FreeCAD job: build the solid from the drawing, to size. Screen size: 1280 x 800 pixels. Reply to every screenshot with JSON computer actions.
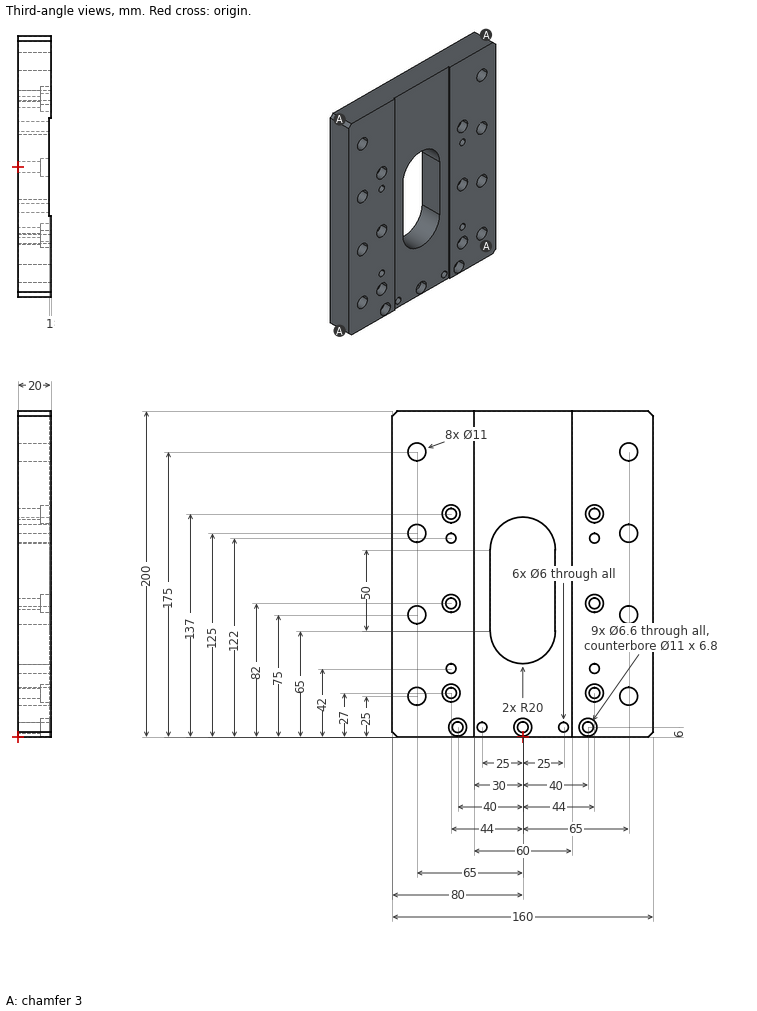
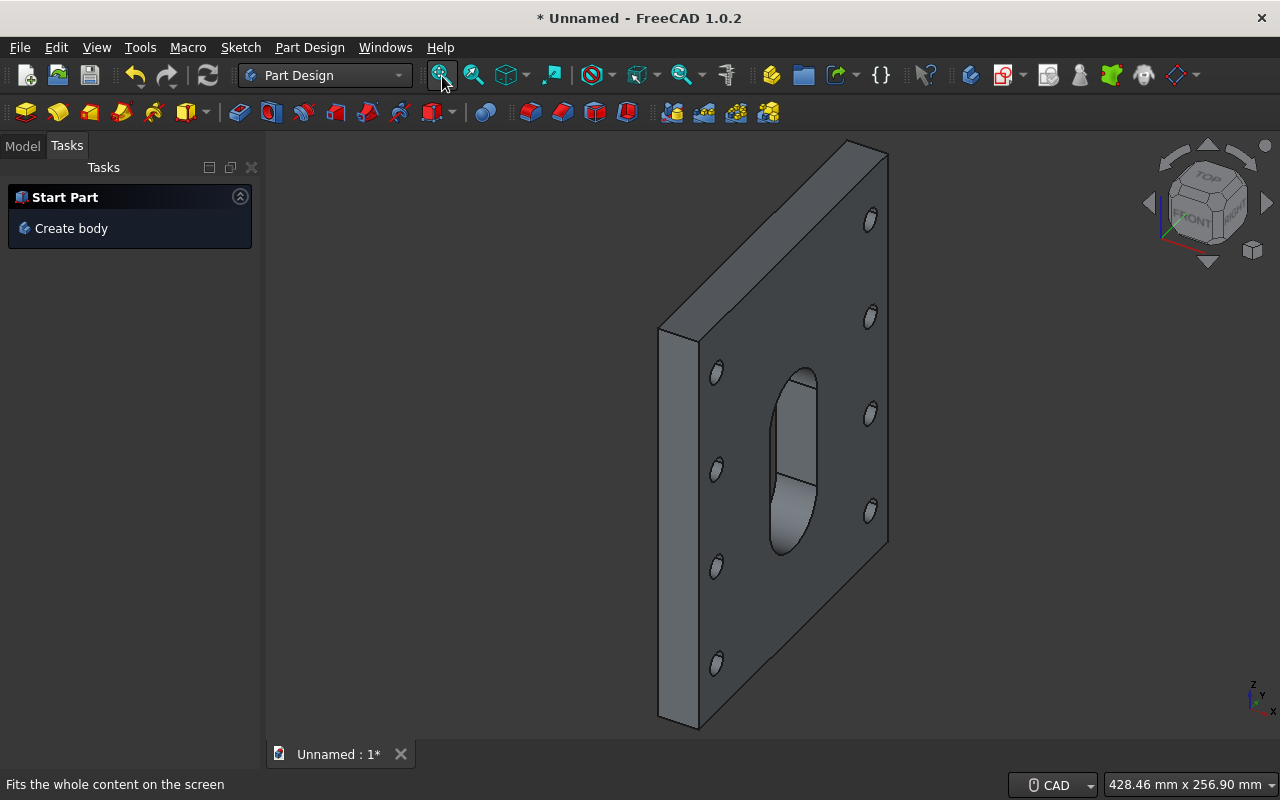
{"action": "left_click", "coordinate": [821, 303]}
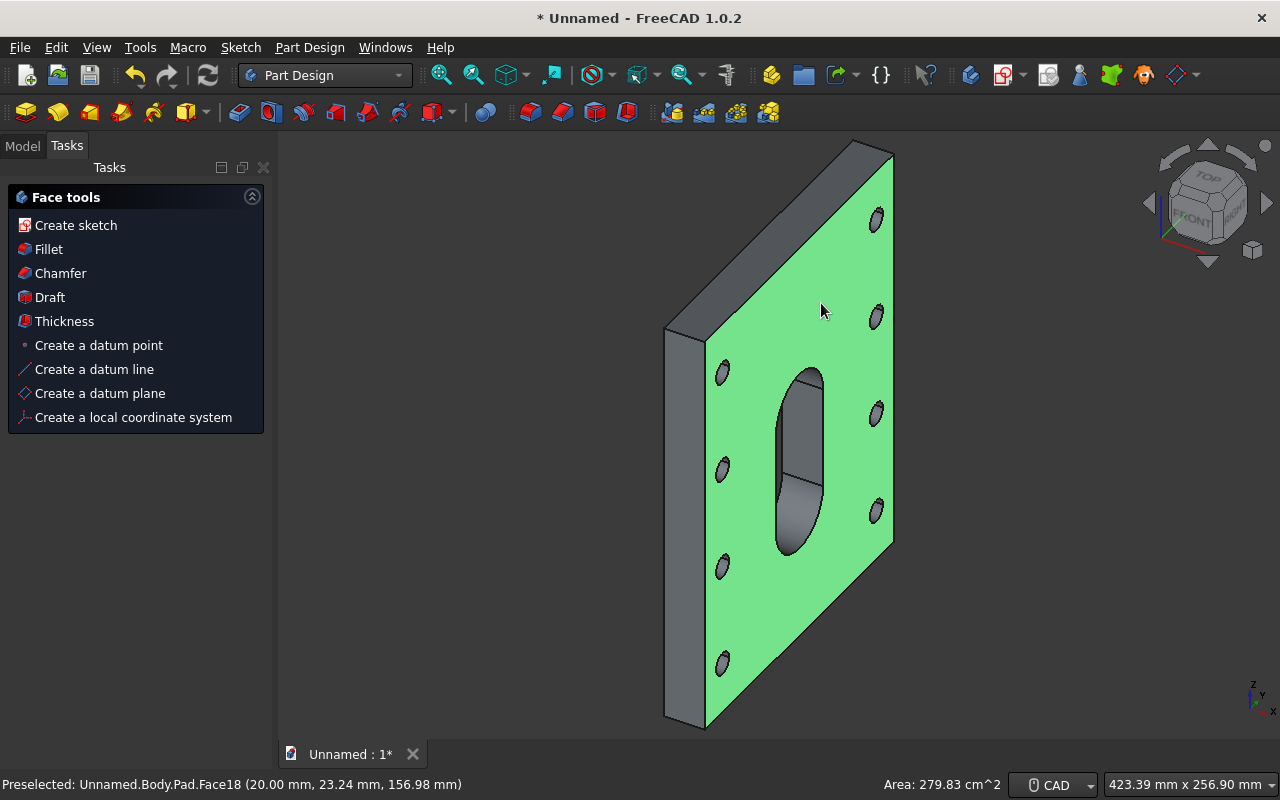
{"action": "left_click", "coordinate": [1004, 76]}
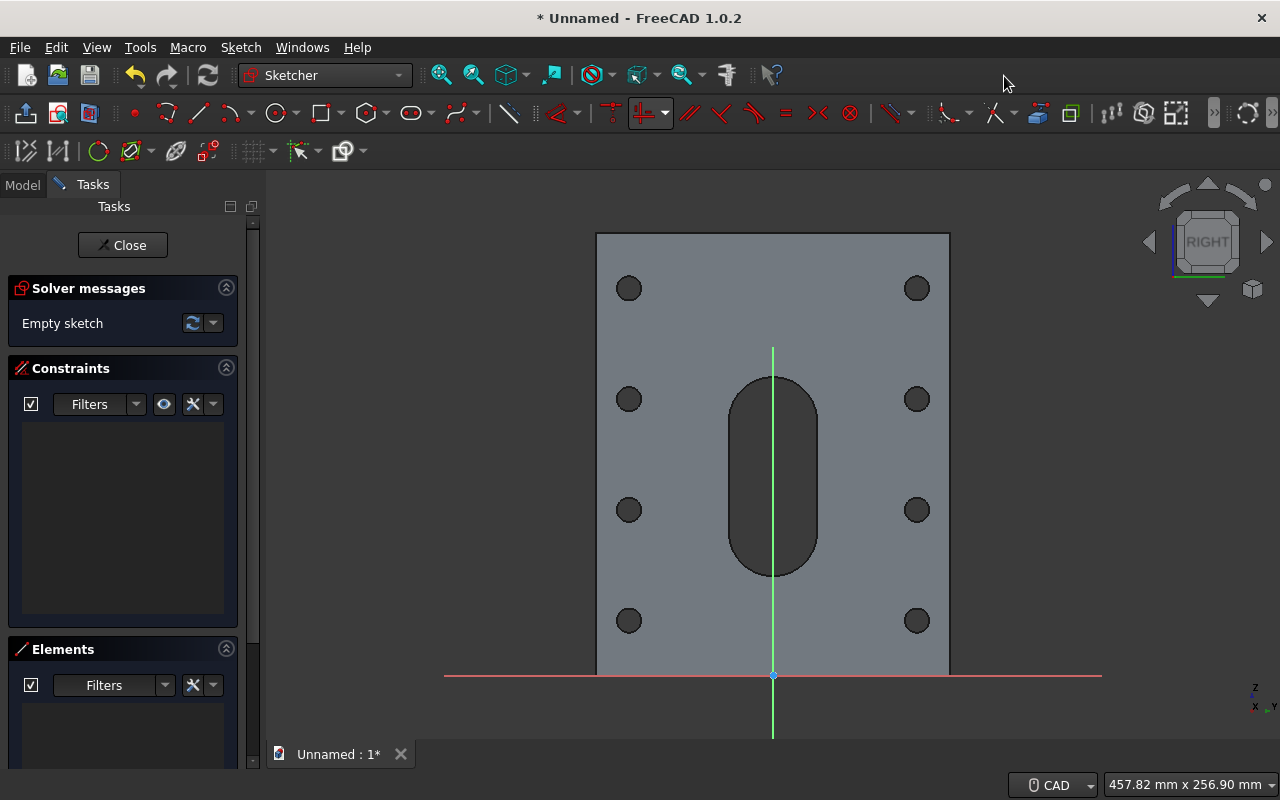
{"action": "key", "text": "g c"}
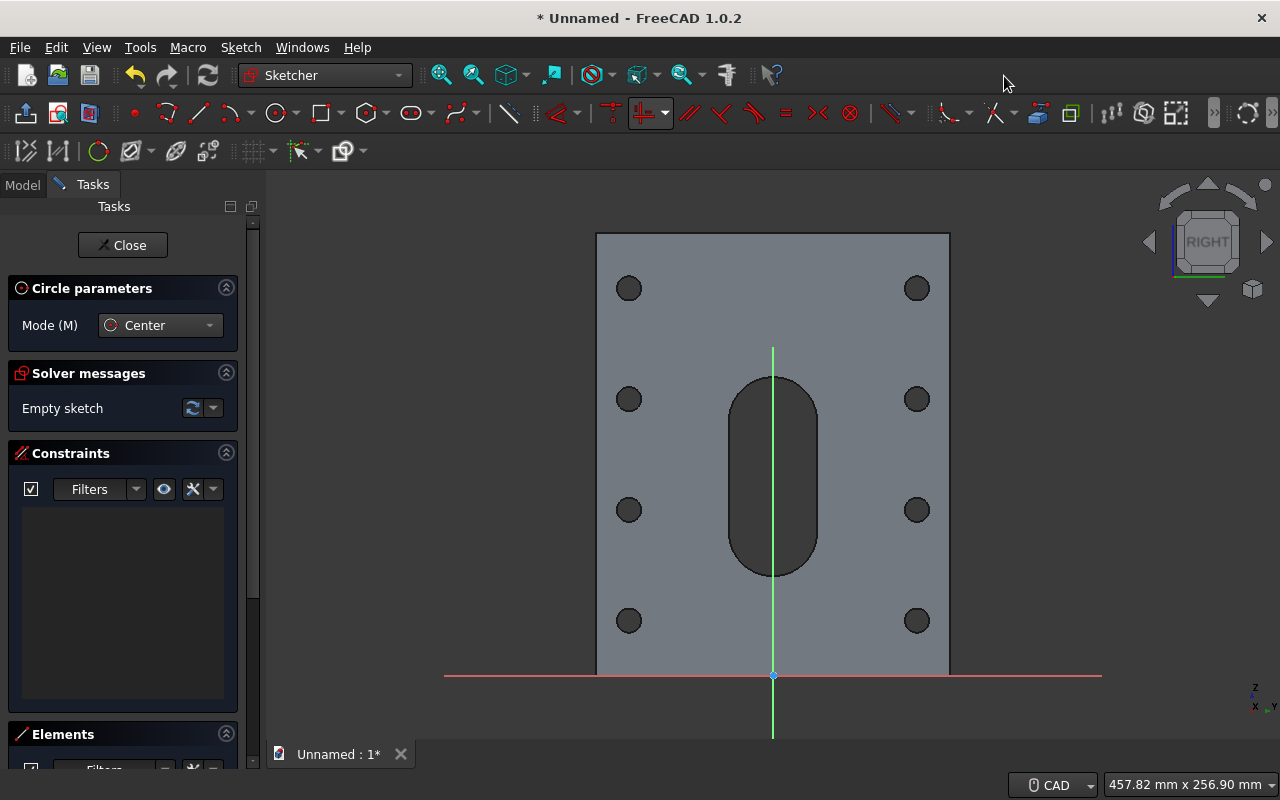
{"action": "scroll", "coordinate": [862, 663], "scroll_direction": "up", "scroll_amount": 6}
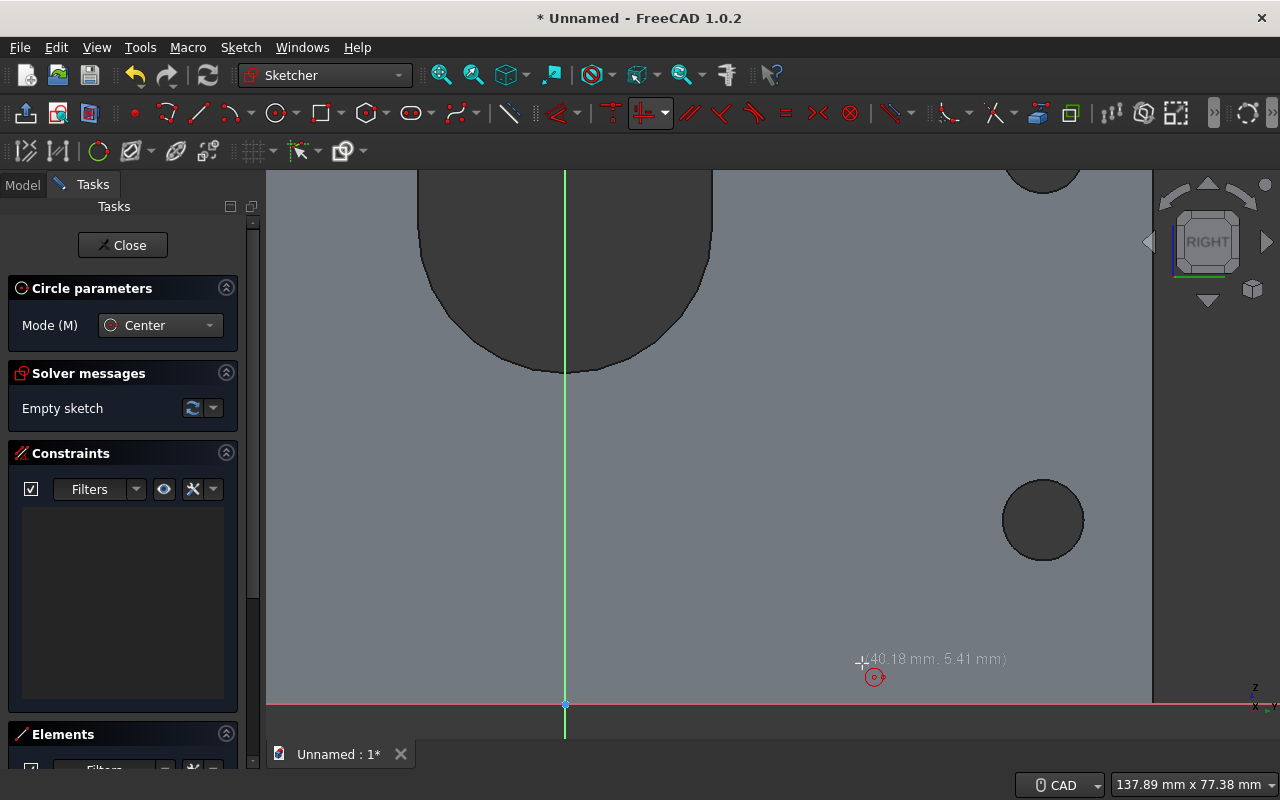
{"action": "left_click", "coordinate": [859, 660]}
{"action": "mouse_move", "coordinate": [876, 643]}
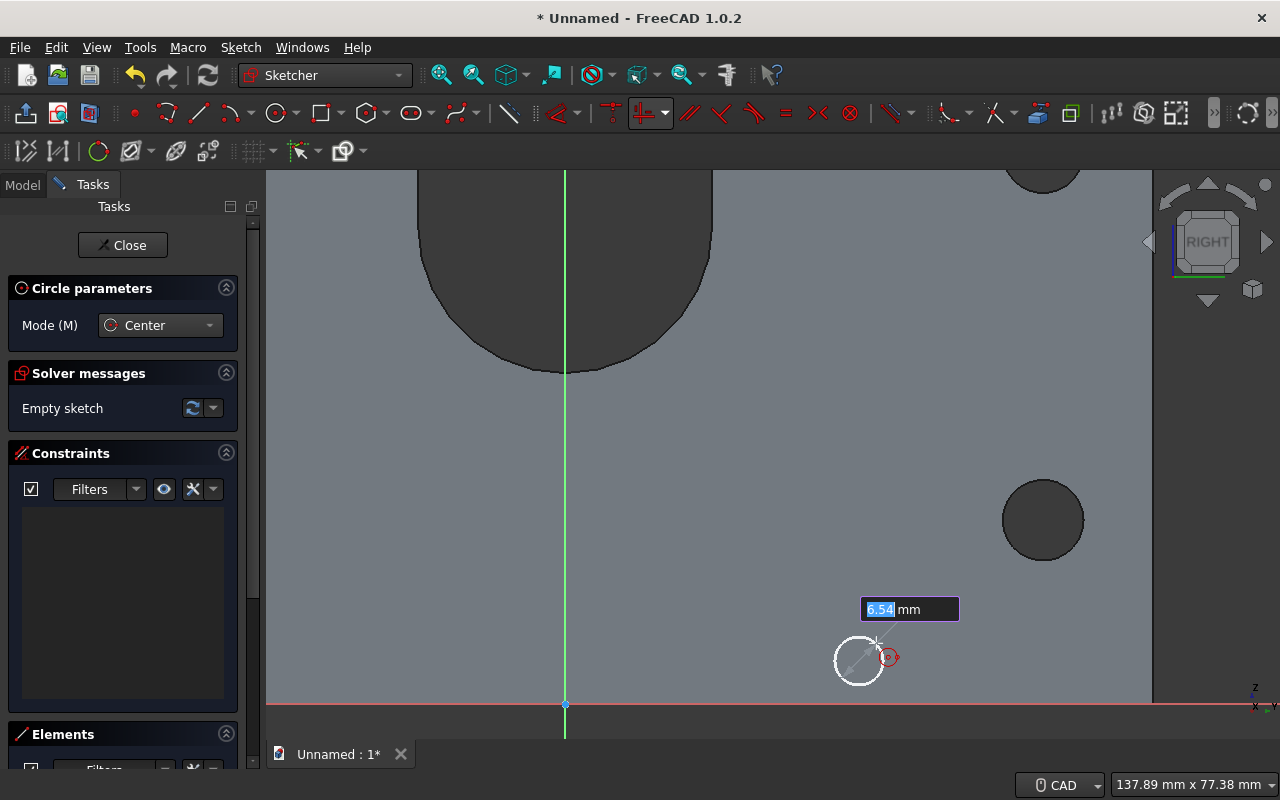
{"action": "type", "text": "6.6"}
{"action": "key", "text": "Return"}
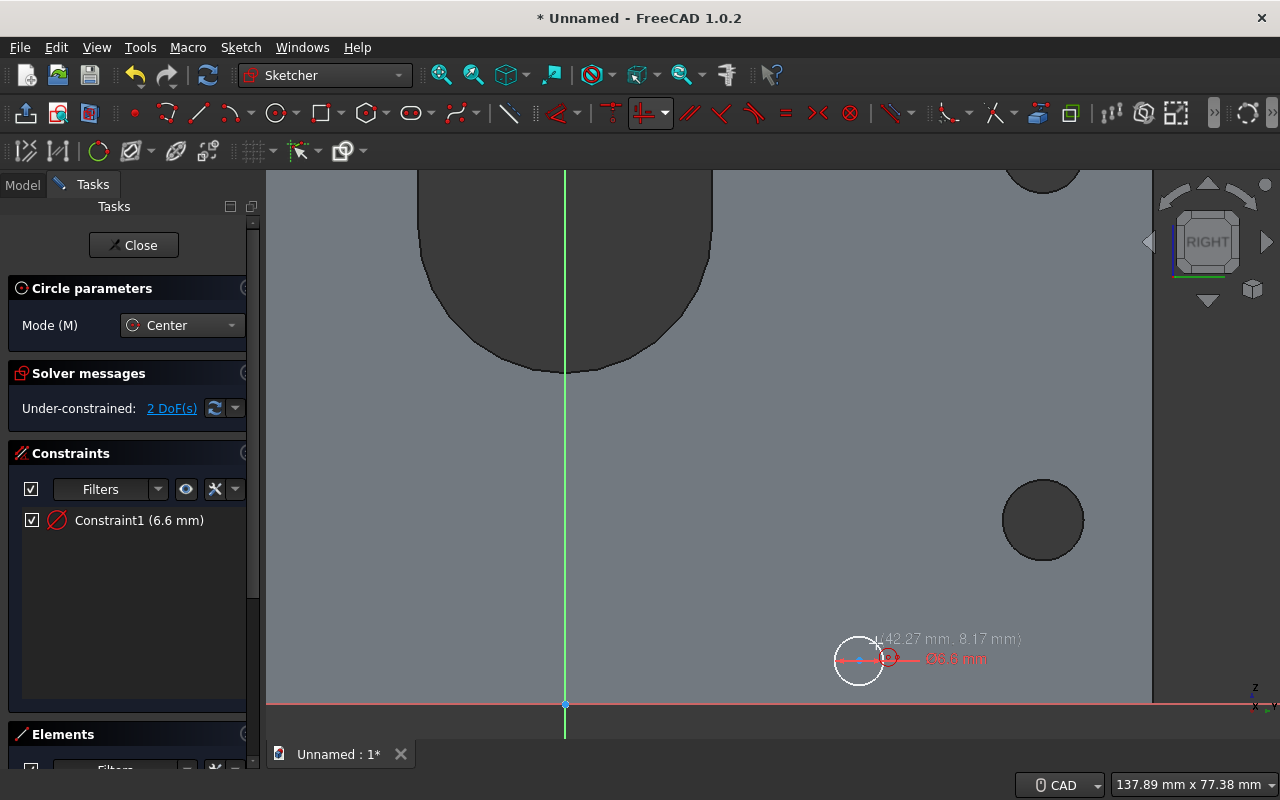
{"action": "left_click", "coordinate": [565, 660]}
{"action": "mouse_move", "coordinate": [582, 643]}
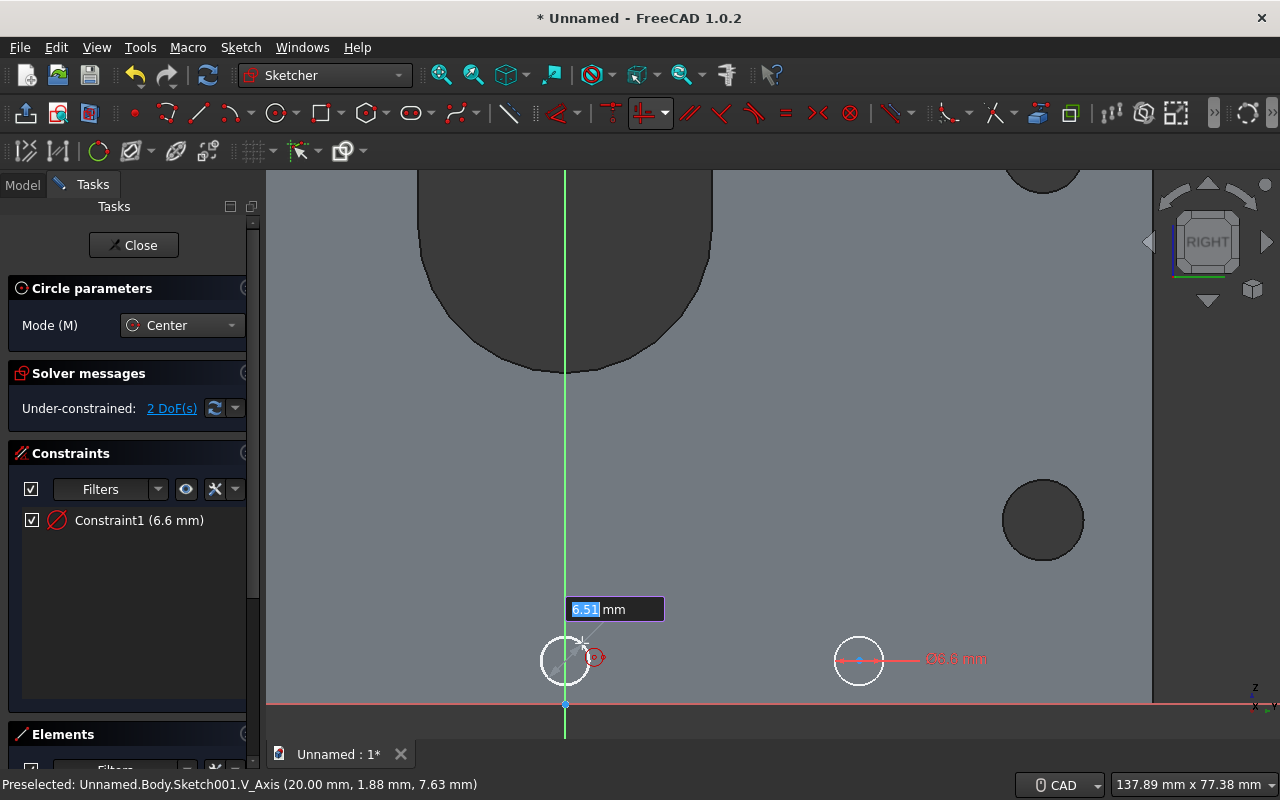
{"action": "type", "text": "6.6"}
{"action": "key", "text": "Return"}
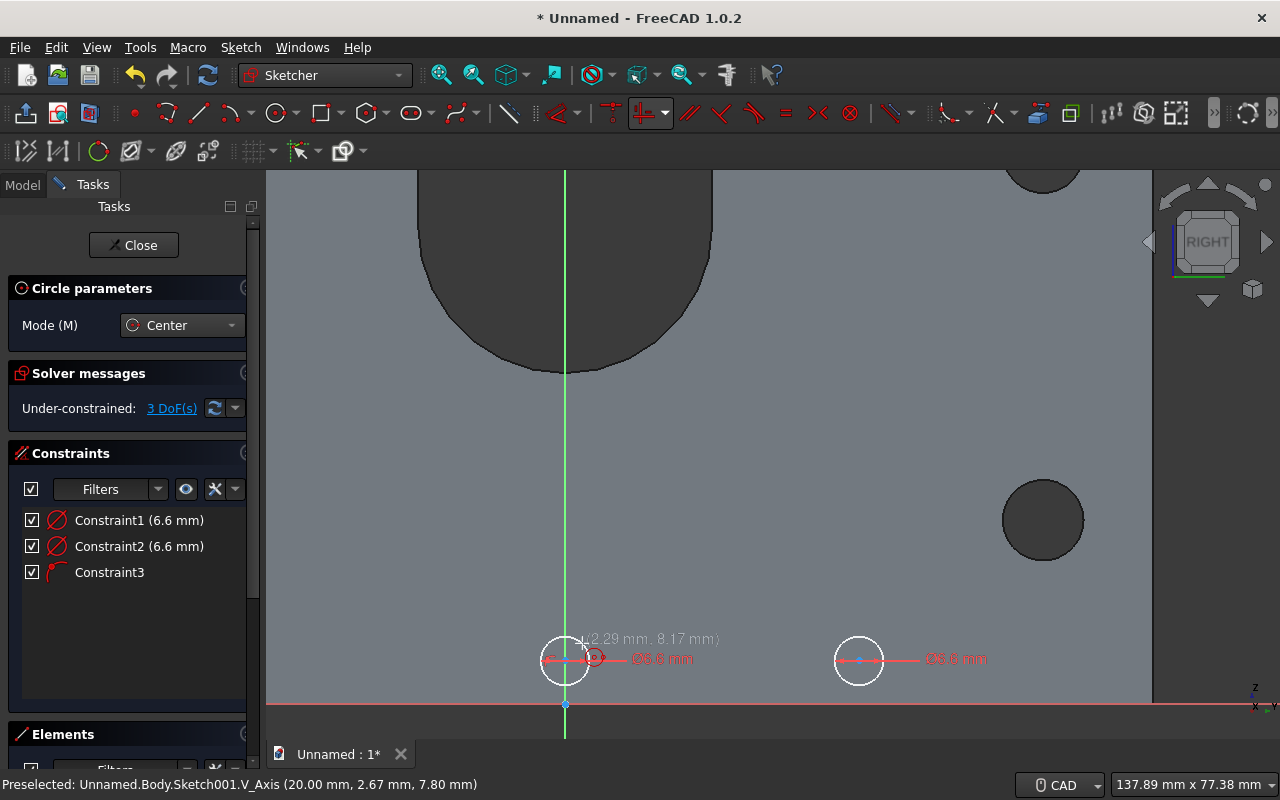
{"action": "scroll", "coordinate": [786, 609], "scroll_direction": "down", "scroll_amount": 5}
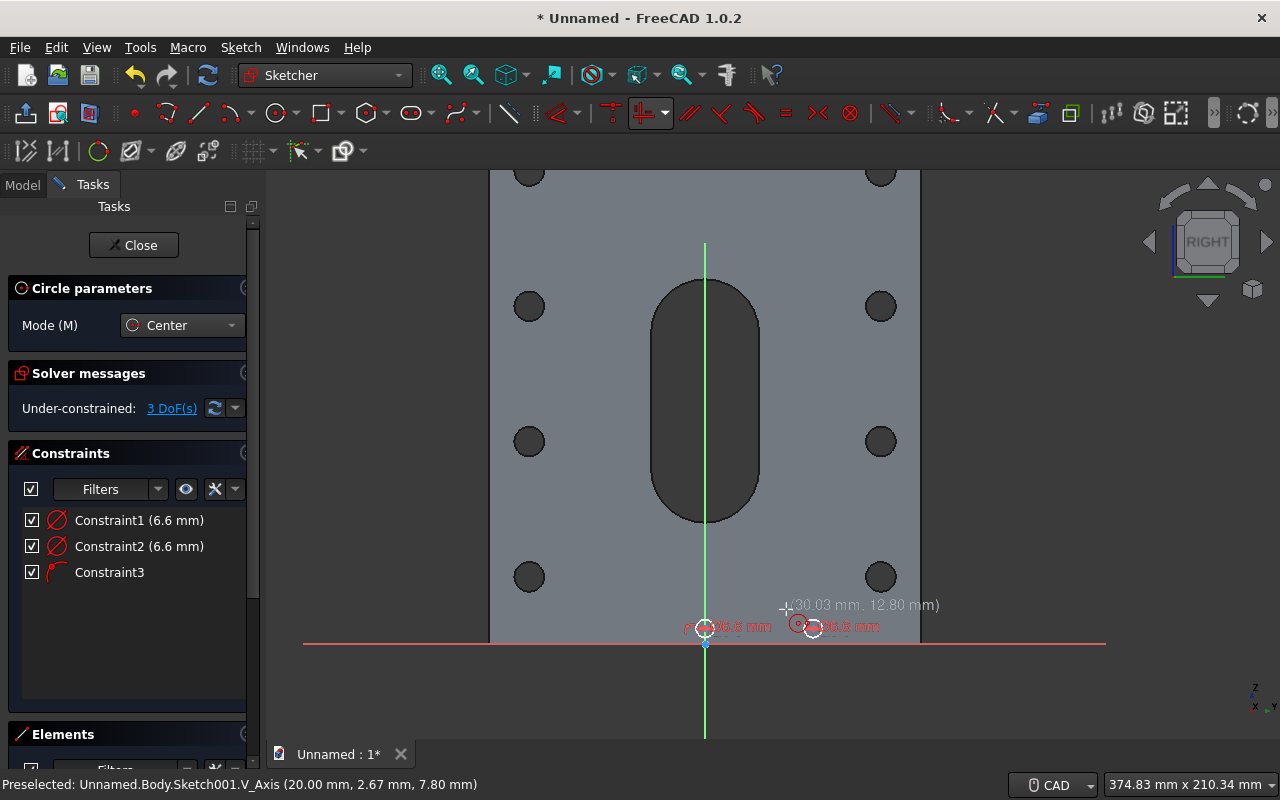
{"action": "scroll", "coordinate": [597, 628], "scroll_direction": "up", "scroll_amount": 5}